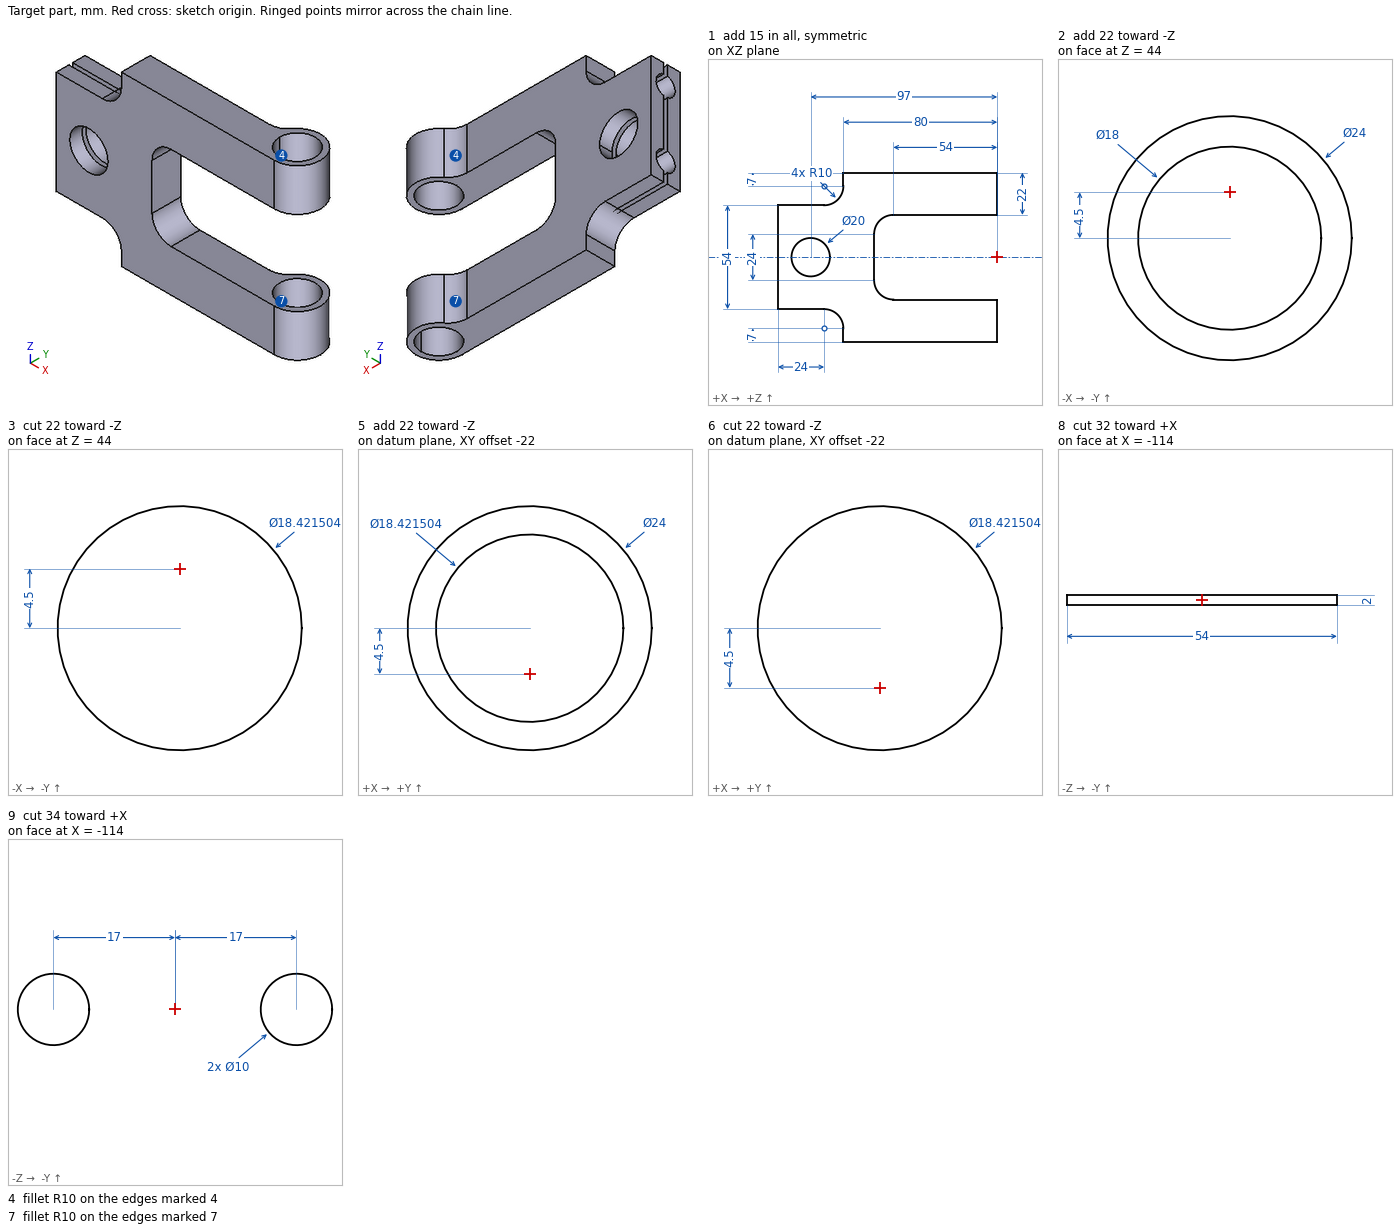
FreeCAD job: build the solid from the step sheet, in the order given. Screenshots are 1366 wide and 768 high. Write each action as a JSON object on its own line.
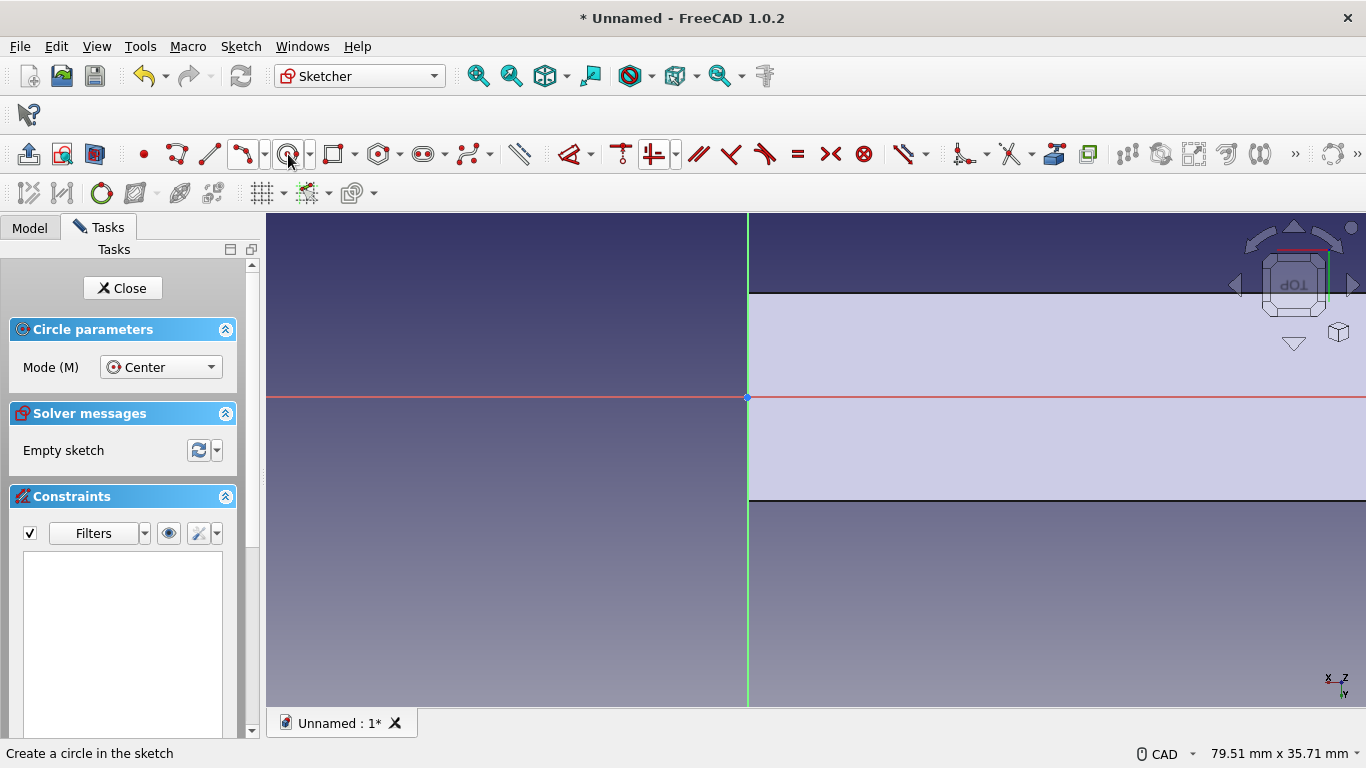
{"action": "left_click", "coordinate": [748, 460]}
{"action": "left_click", "coordinate": [865, 342]}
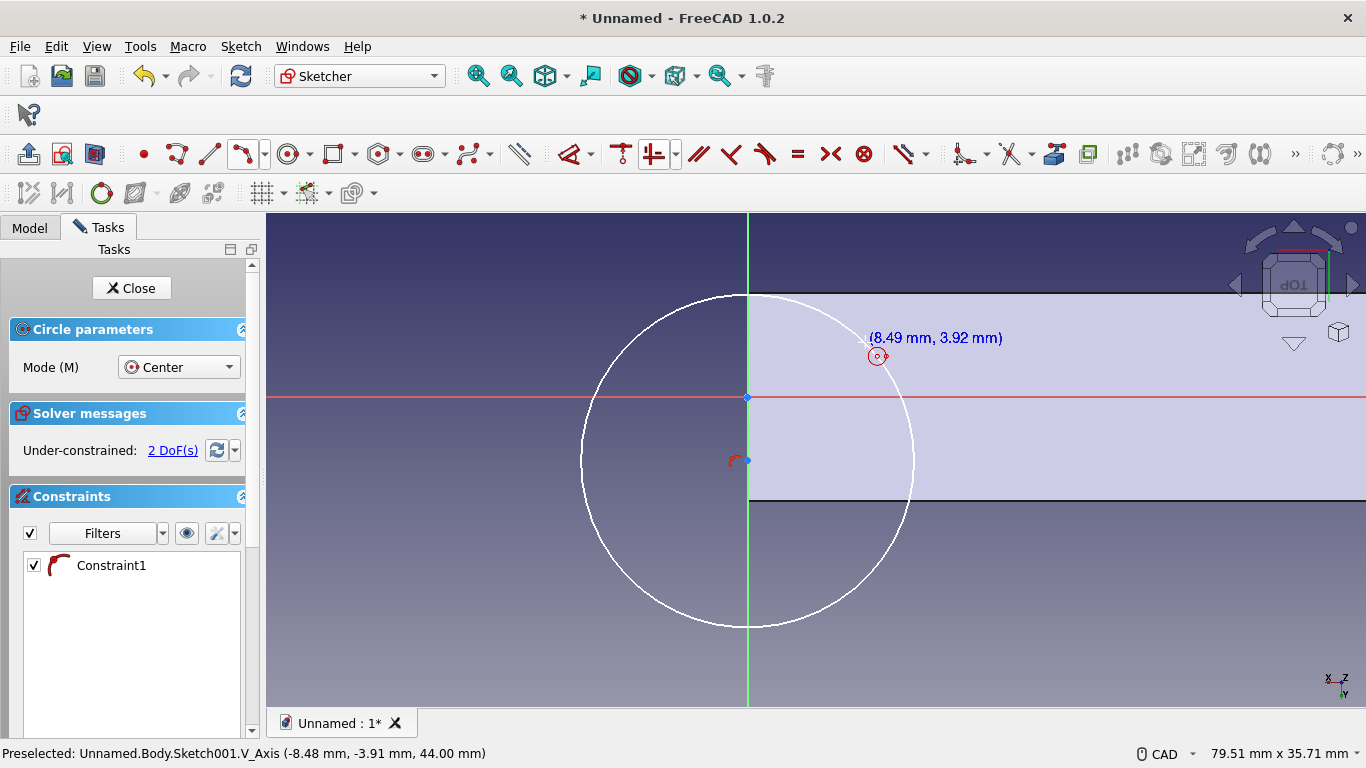
{"action": "left_click", "coordinate": [748, 461]}
{"action": "left_click", "coordinate": [836, 371]}
{"action": "key", "text": "Escape"}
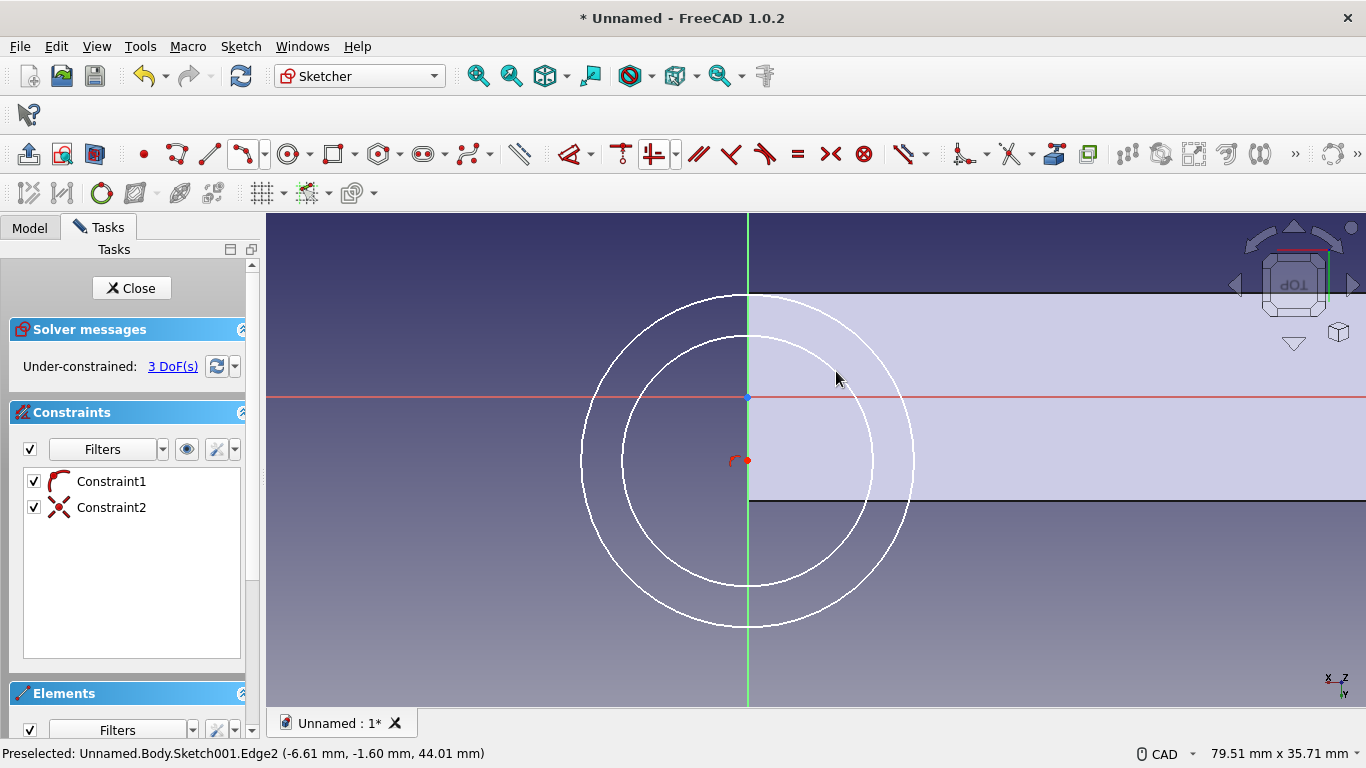
{"action": "left_click", "coordinate": [568, 154]}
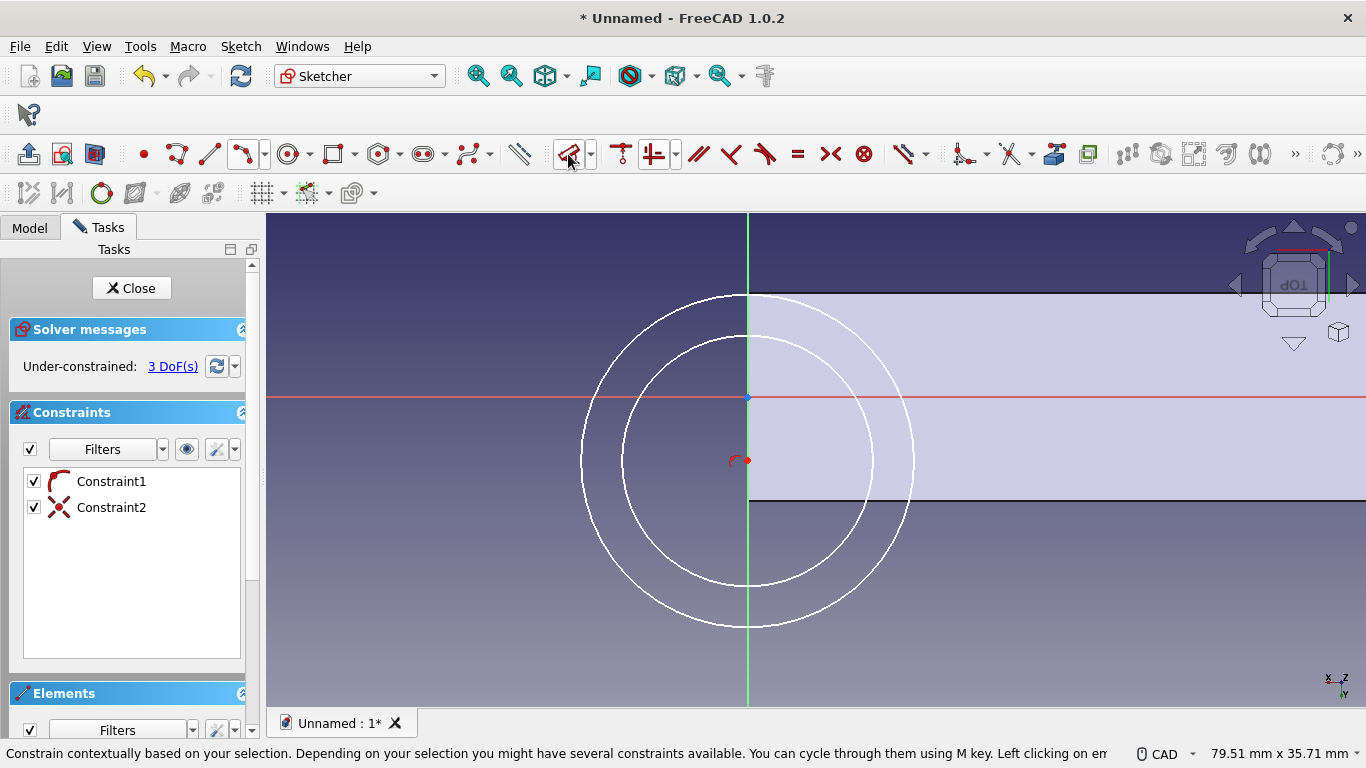
{"action": "left_click", "coordinate": [865, 343]}
{"action": "left_click", "coordinate": [888, 320]}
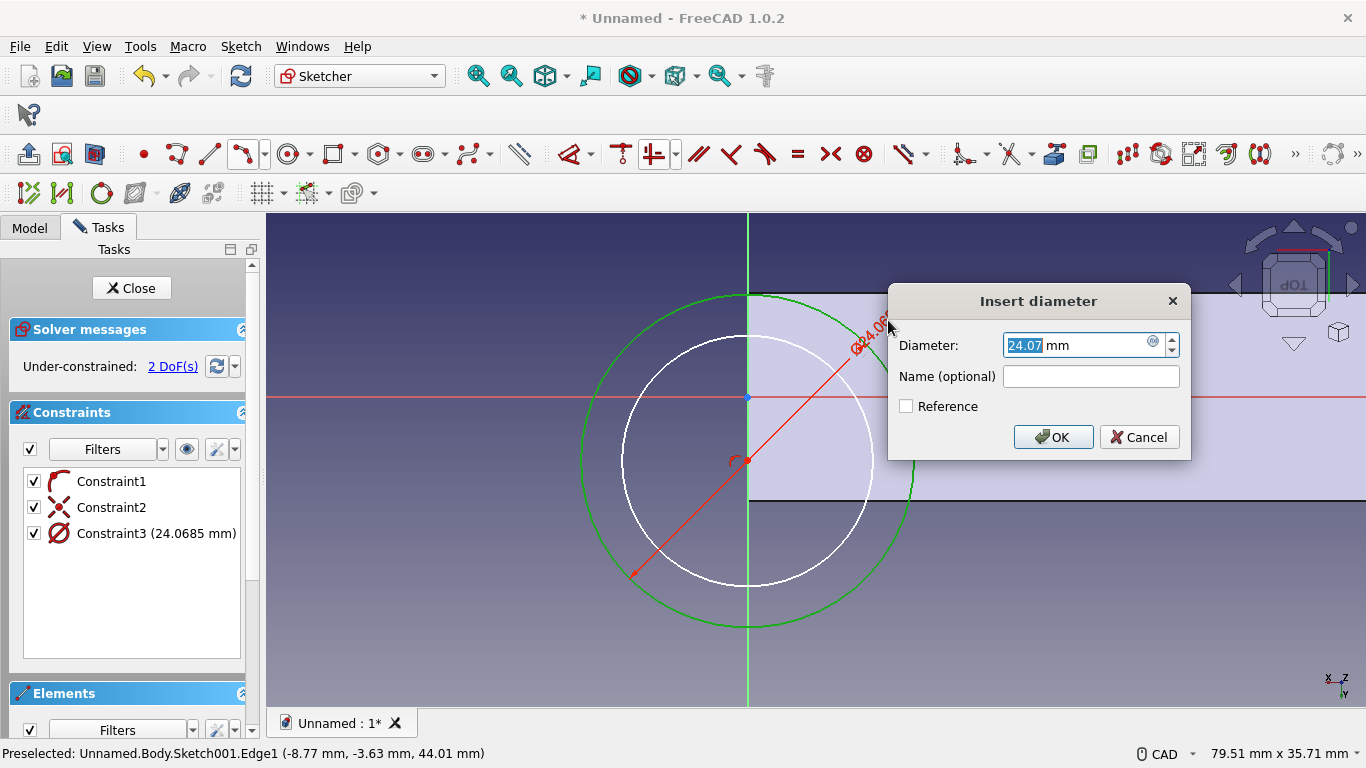
{"action": "type", "text": "24"}
{"action": "key", "text": "Return"}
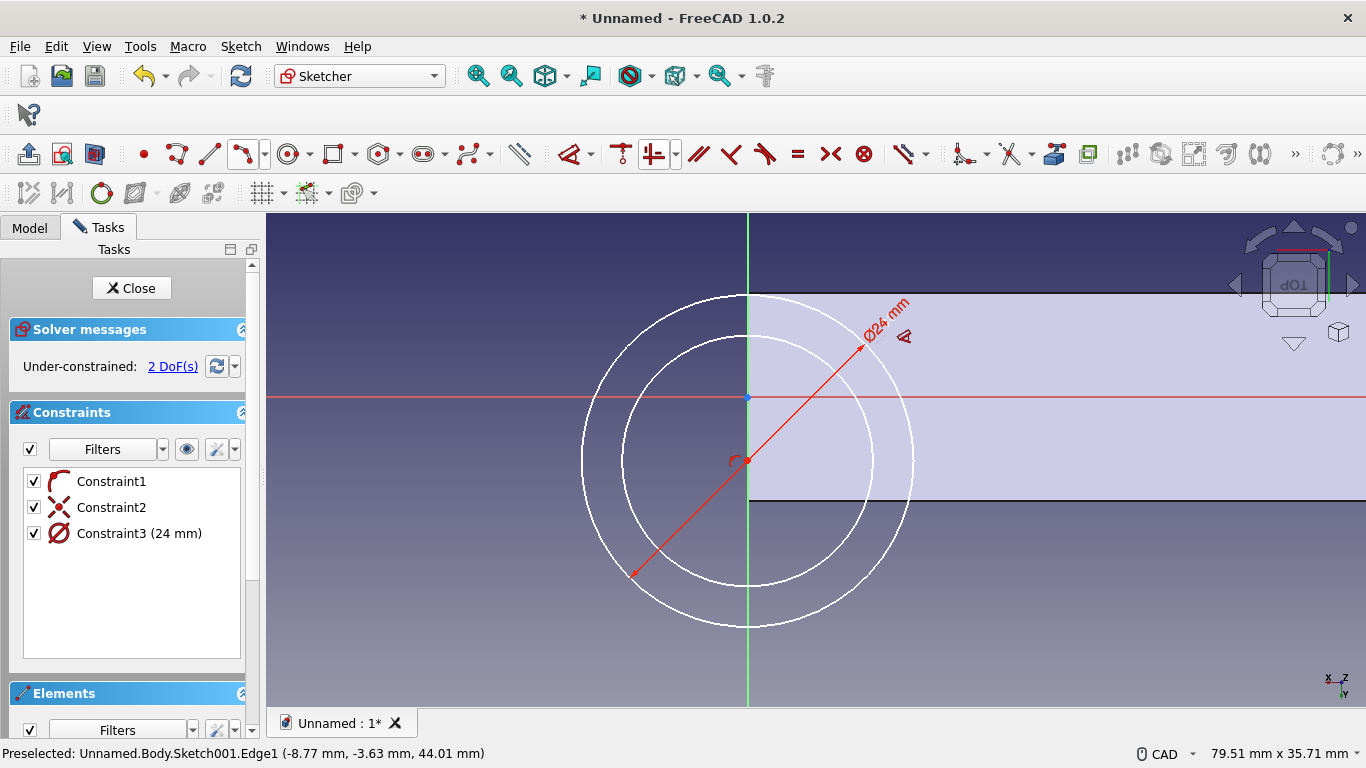
{"action": "left_click", "coordinate": [836, 372]}
{"action": "left_click", "coordinate": [798, 288]}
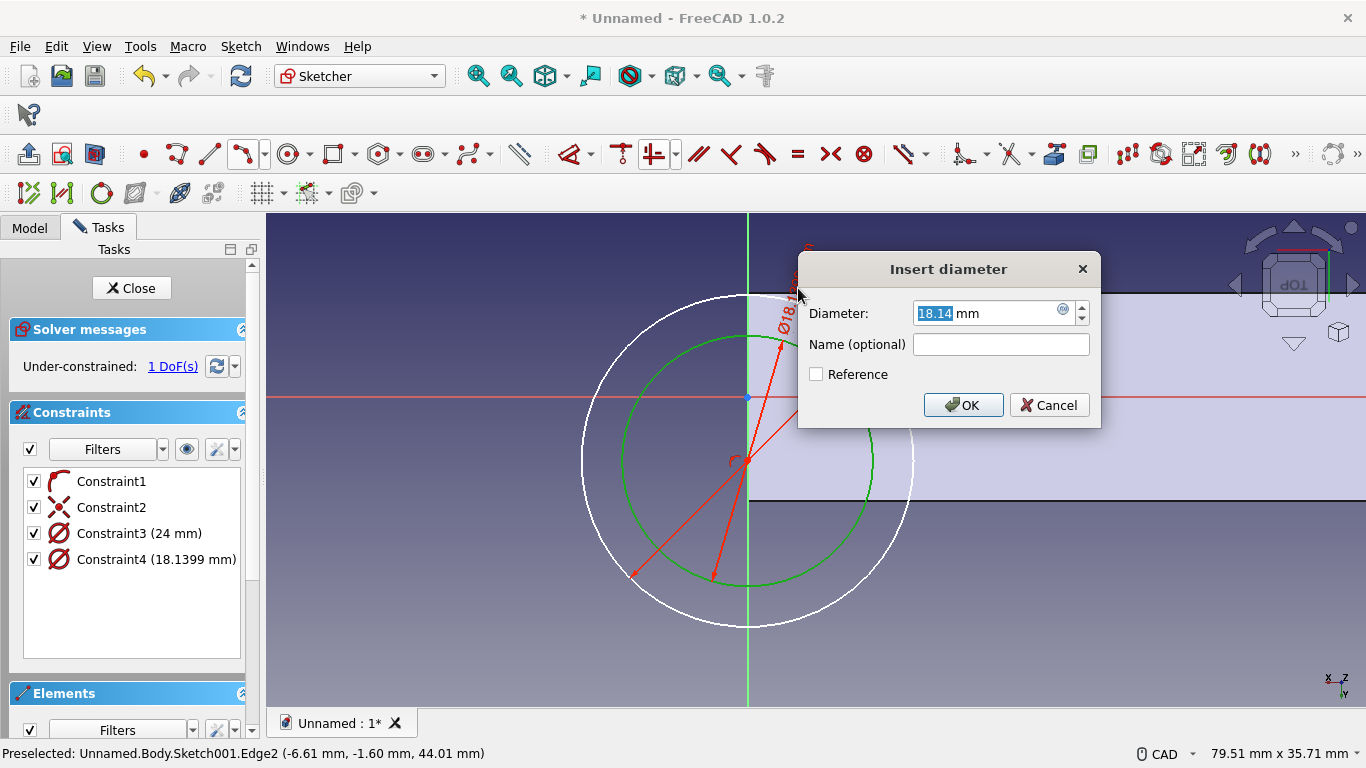
{"action": "type", "text": "18"}
{"action": "key", "text": "Return"}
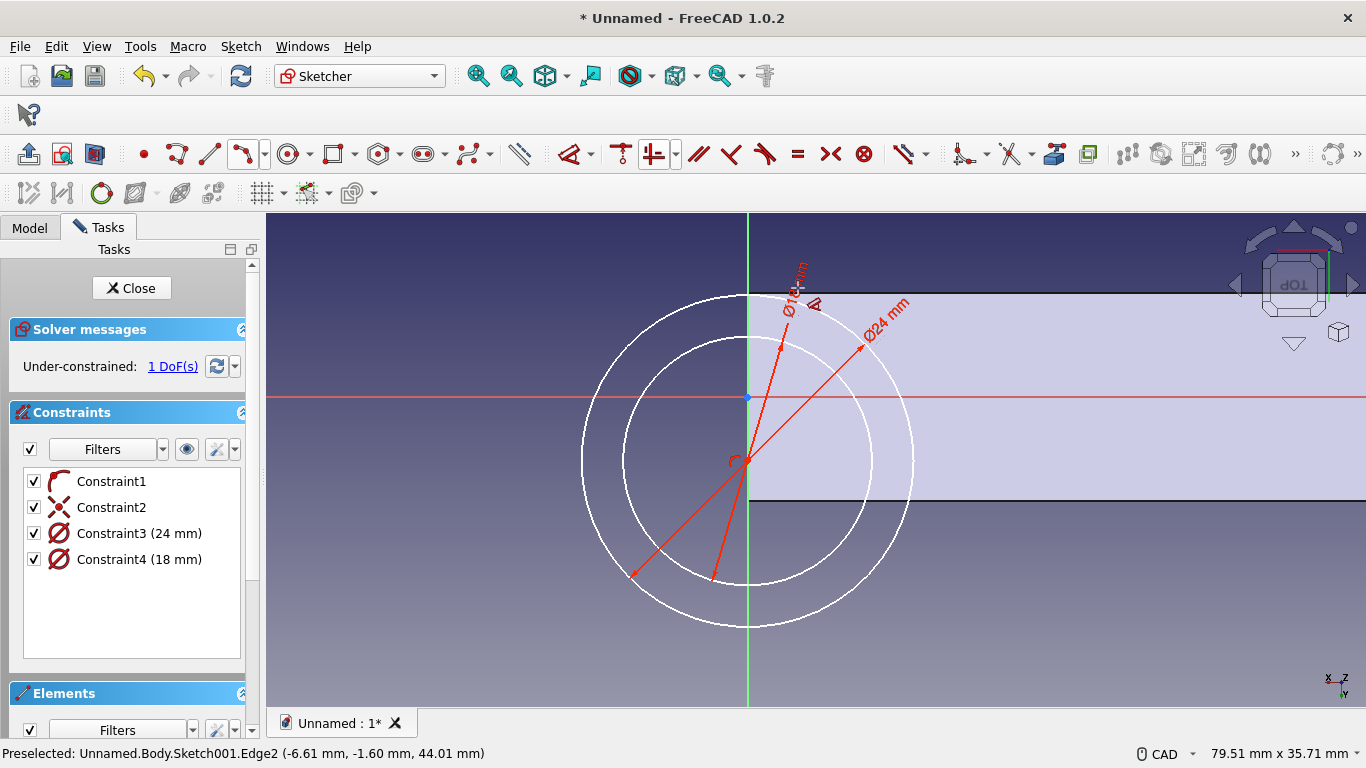
{"action": "left_click", "coordinate": [748, 461]}
{"action": "left_click", "coordinate": [782, 429]}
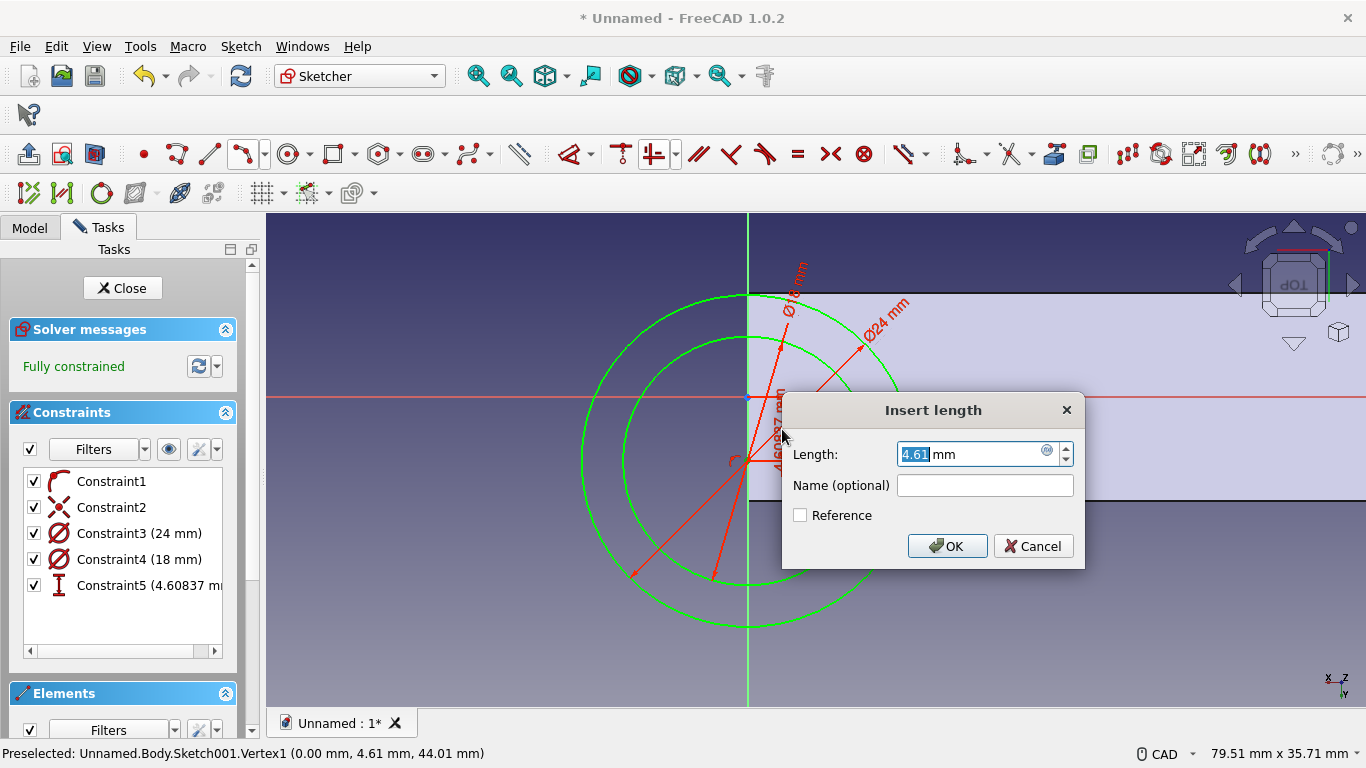
{"action": "type", "text": "4.5"}
{"action": "key", "text": "Return"}
{"action": "key", "text": "Escape"}